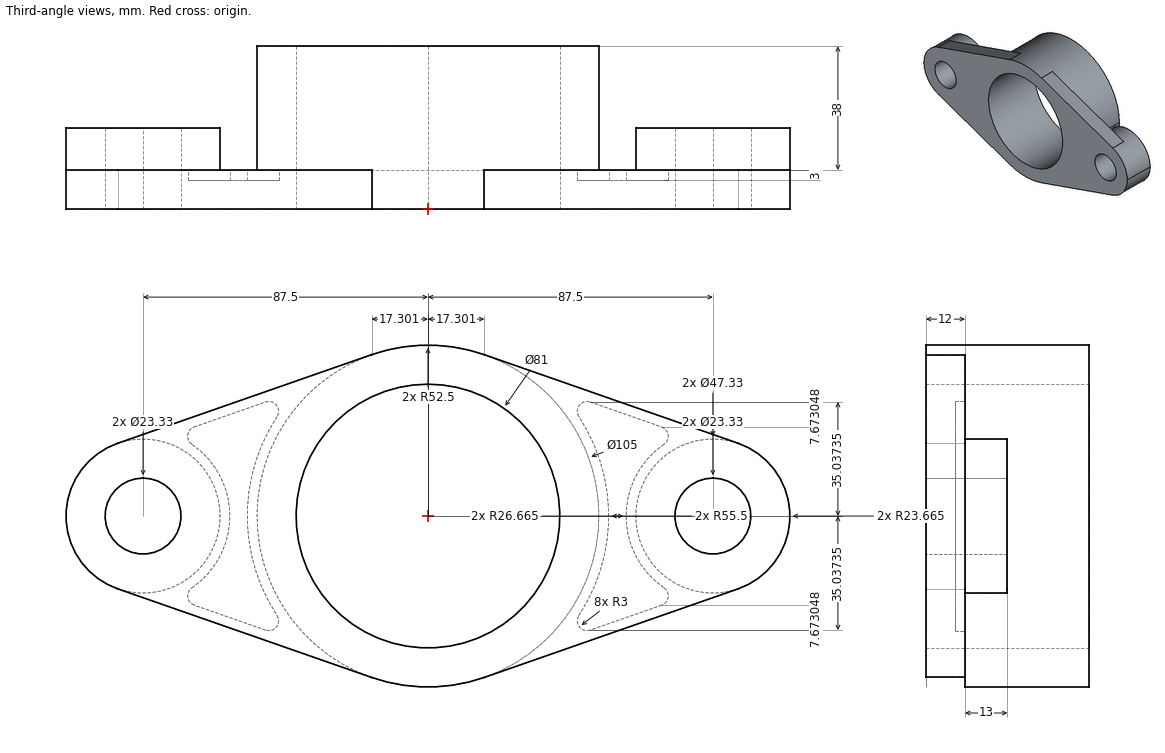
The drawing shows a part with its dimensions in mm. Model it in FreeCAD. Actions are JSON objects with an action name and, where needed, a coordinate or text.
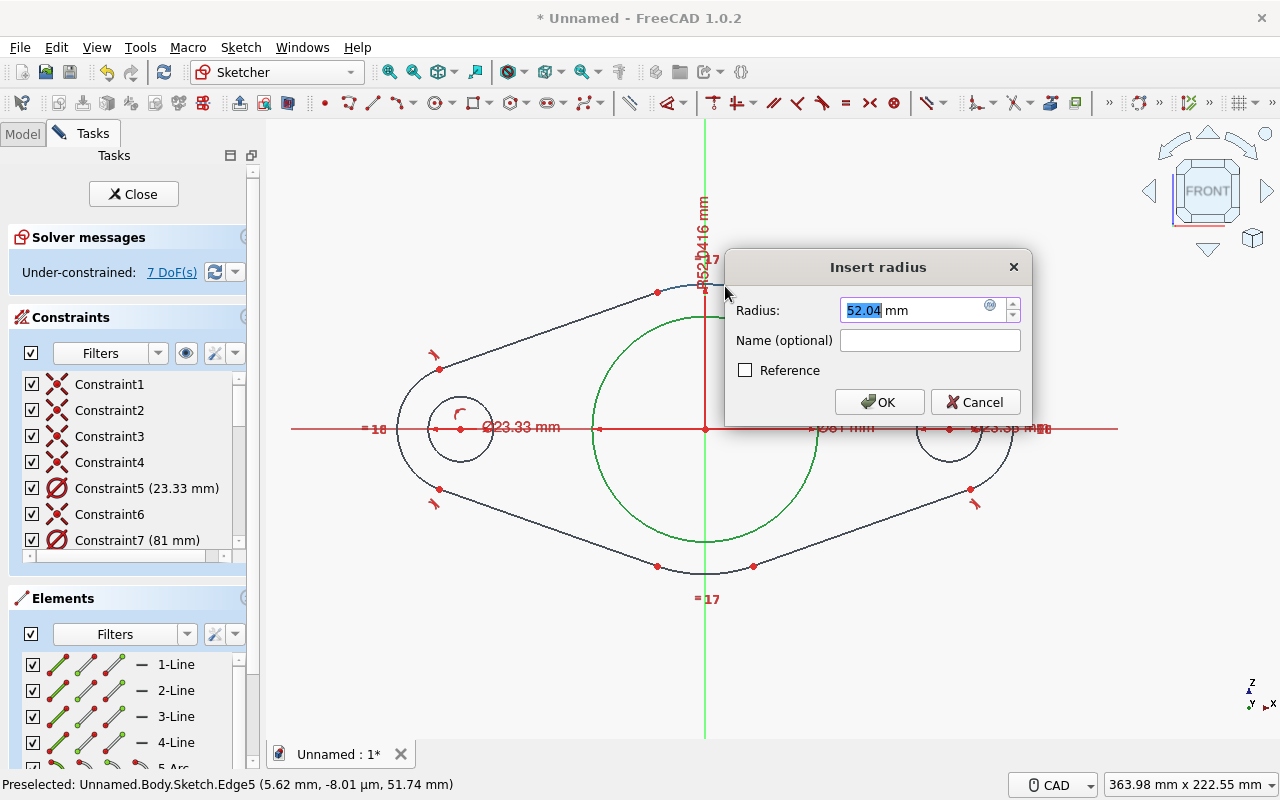
{"action": "type", "text": "52.5"}
{"action": "key", "text": "Return"}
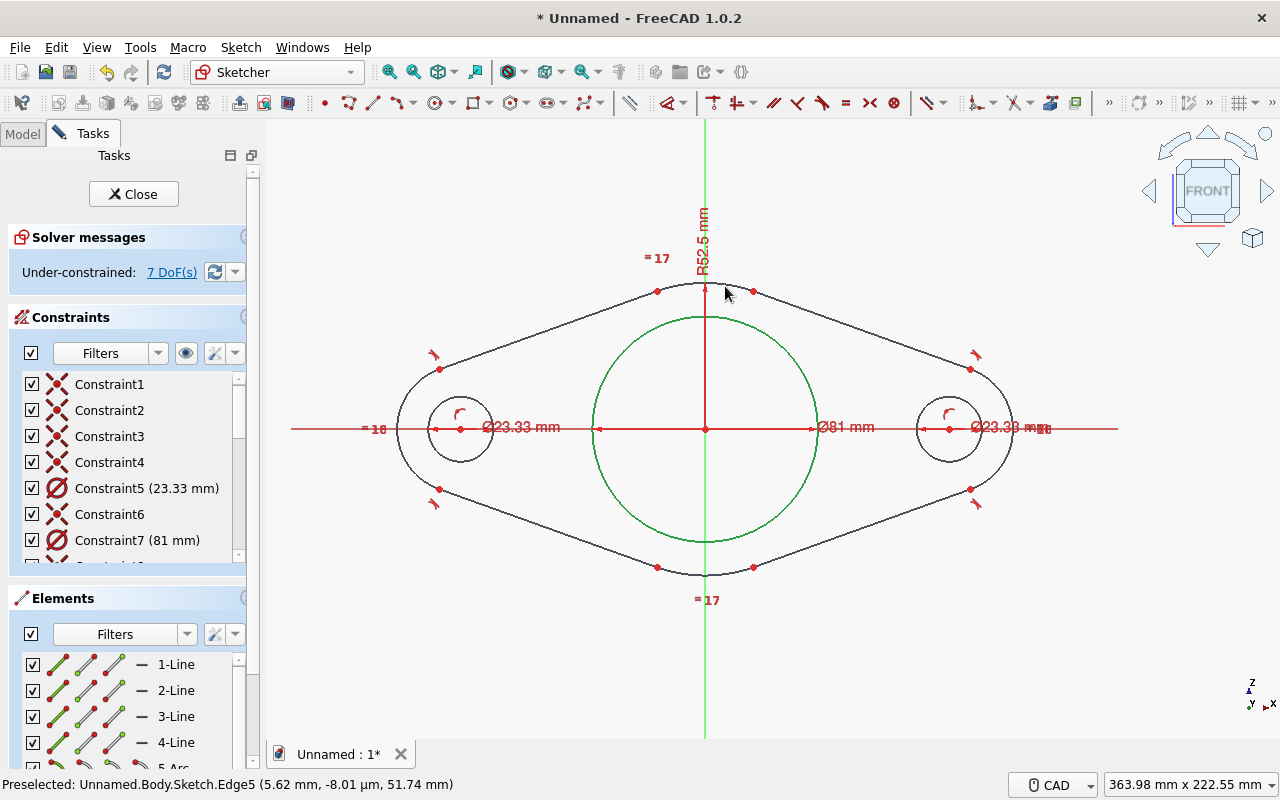
{"action": "left_click", "coordinate": [1005, 459]}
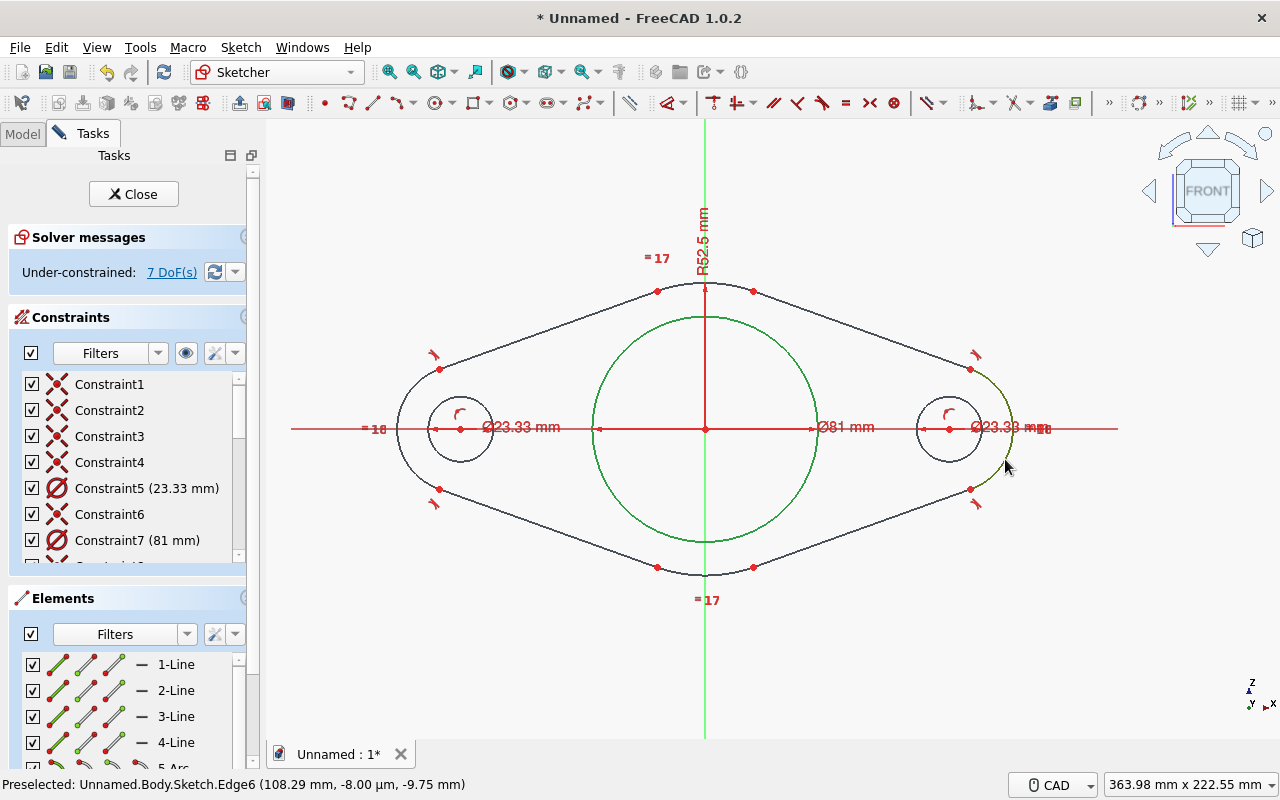
{"action": "left_click", "coordinate": [686, 104]}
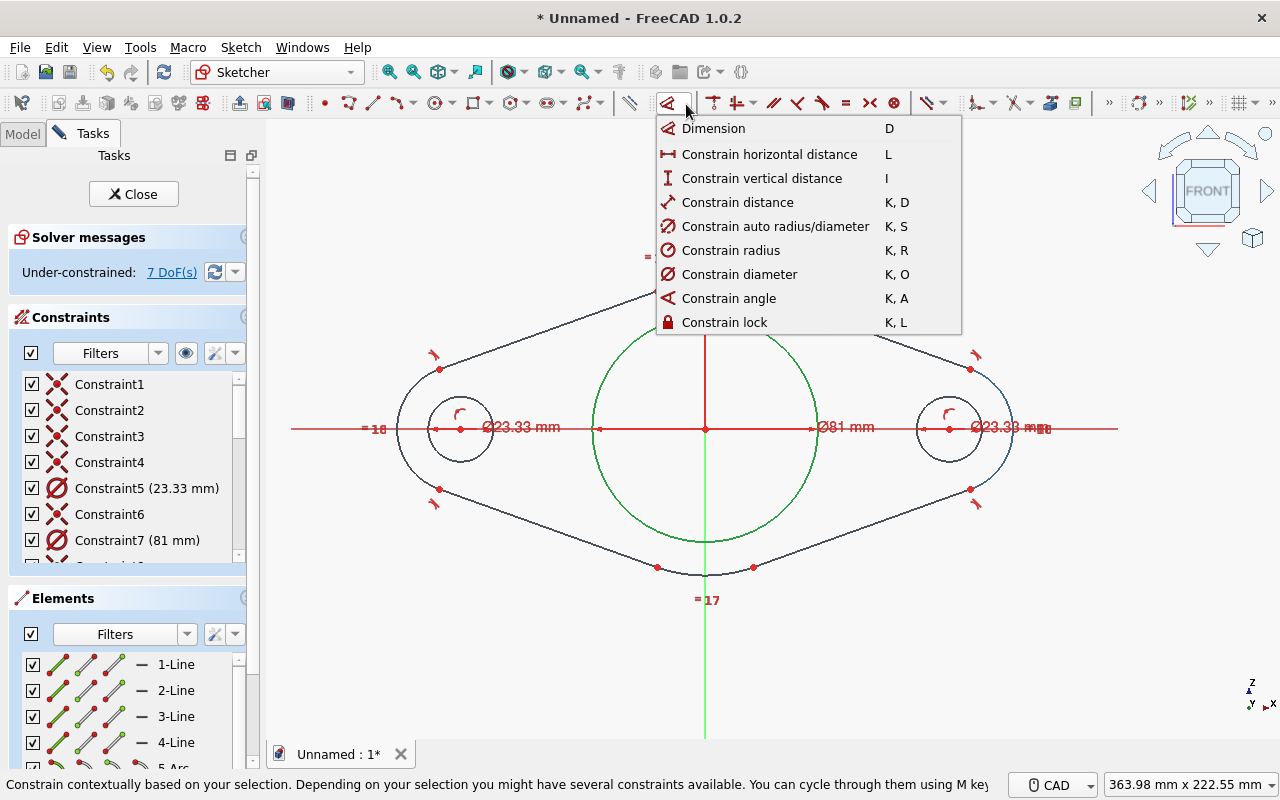
{"action": "left_click", "coordinate": [809, 250]}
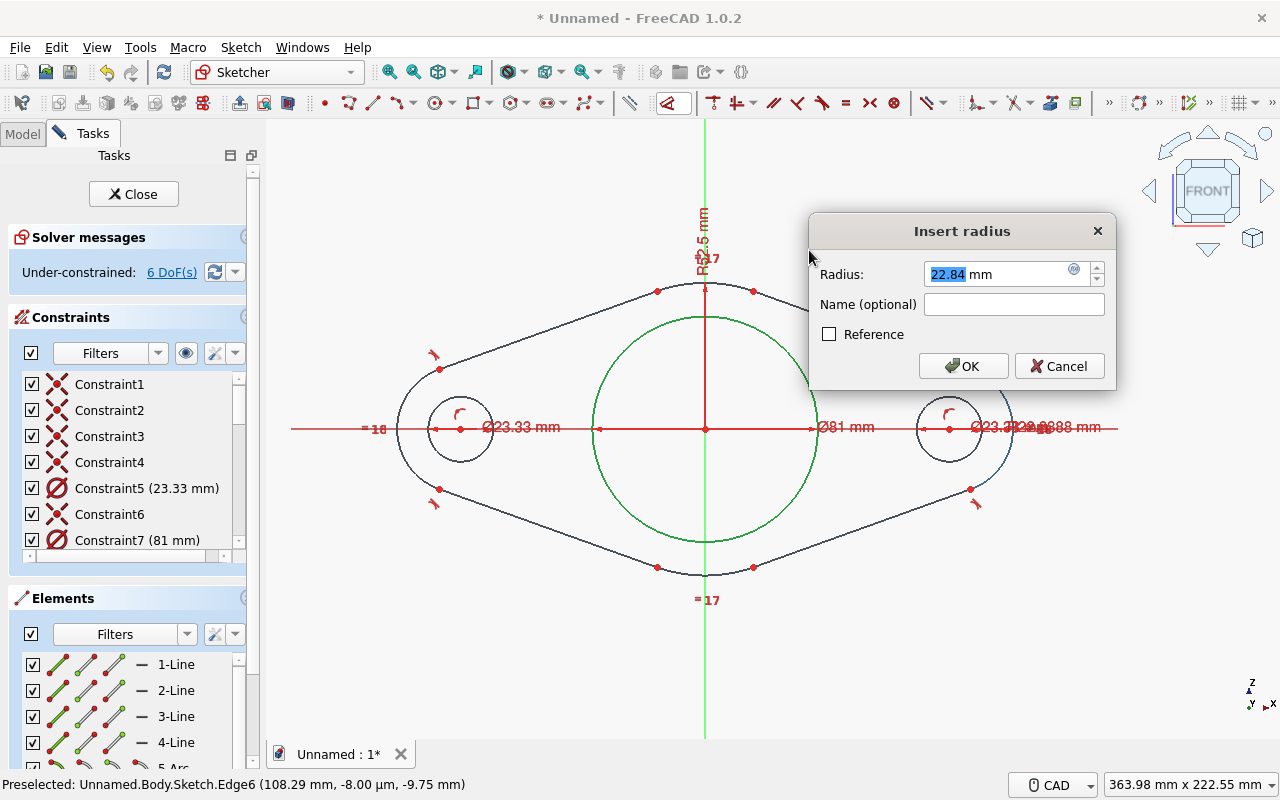
{"action": "type", "text": "23.665"}
{"action": "key", "text": "Return"}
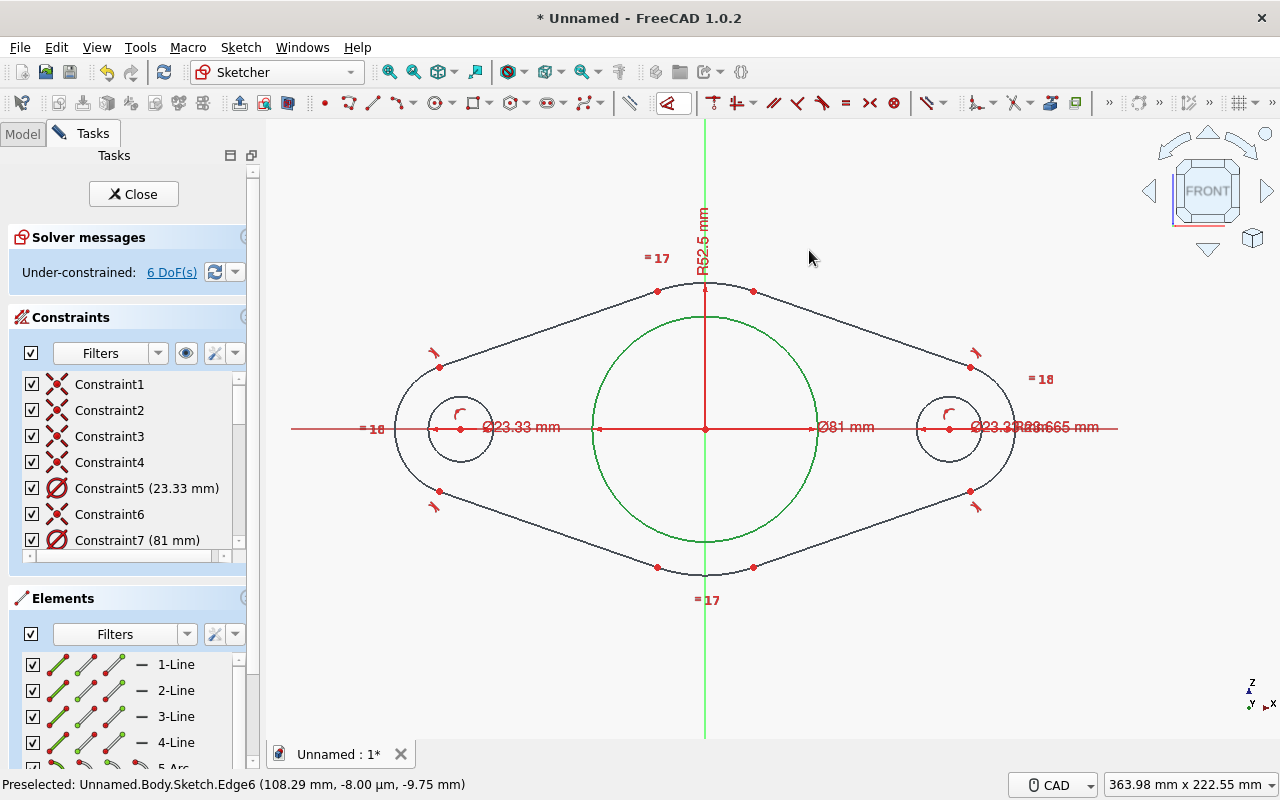
{"action": "left_click", "coordinate": [461, 429]}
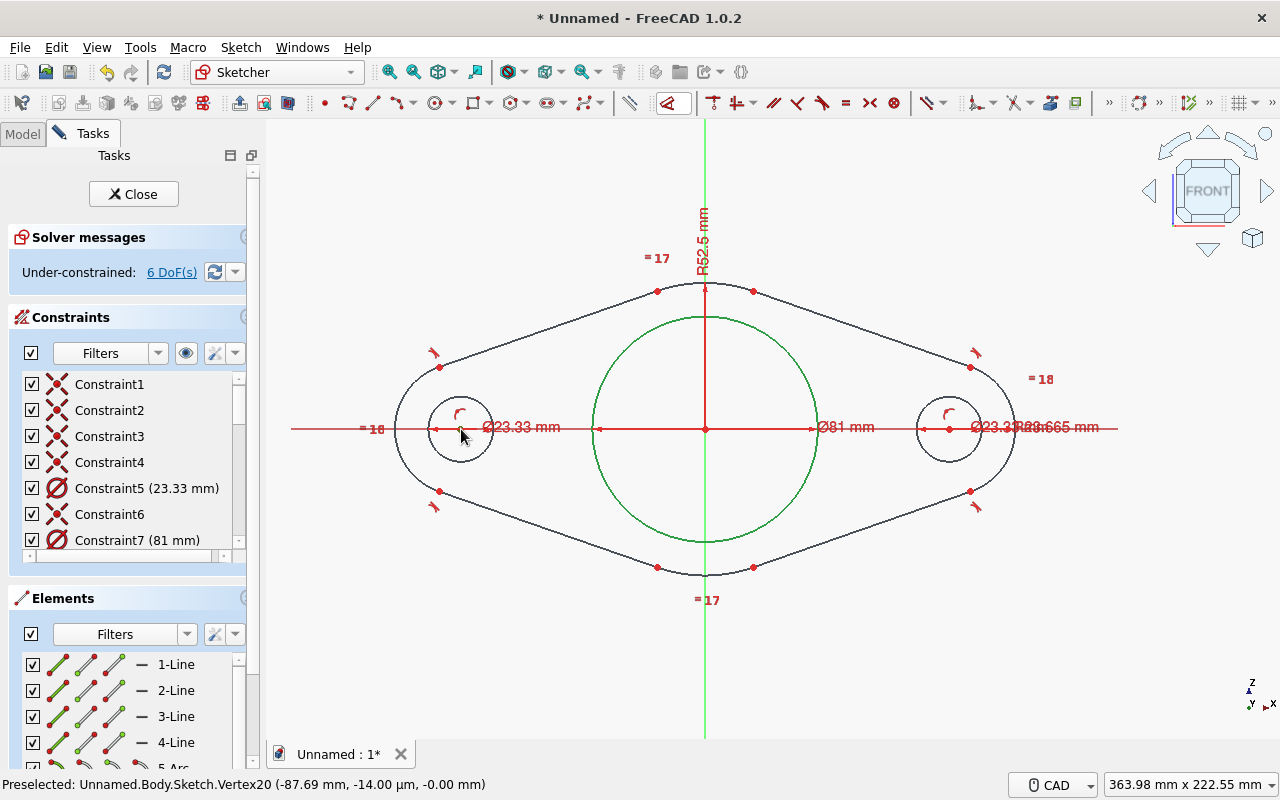
{"action": "key", "text": "l"}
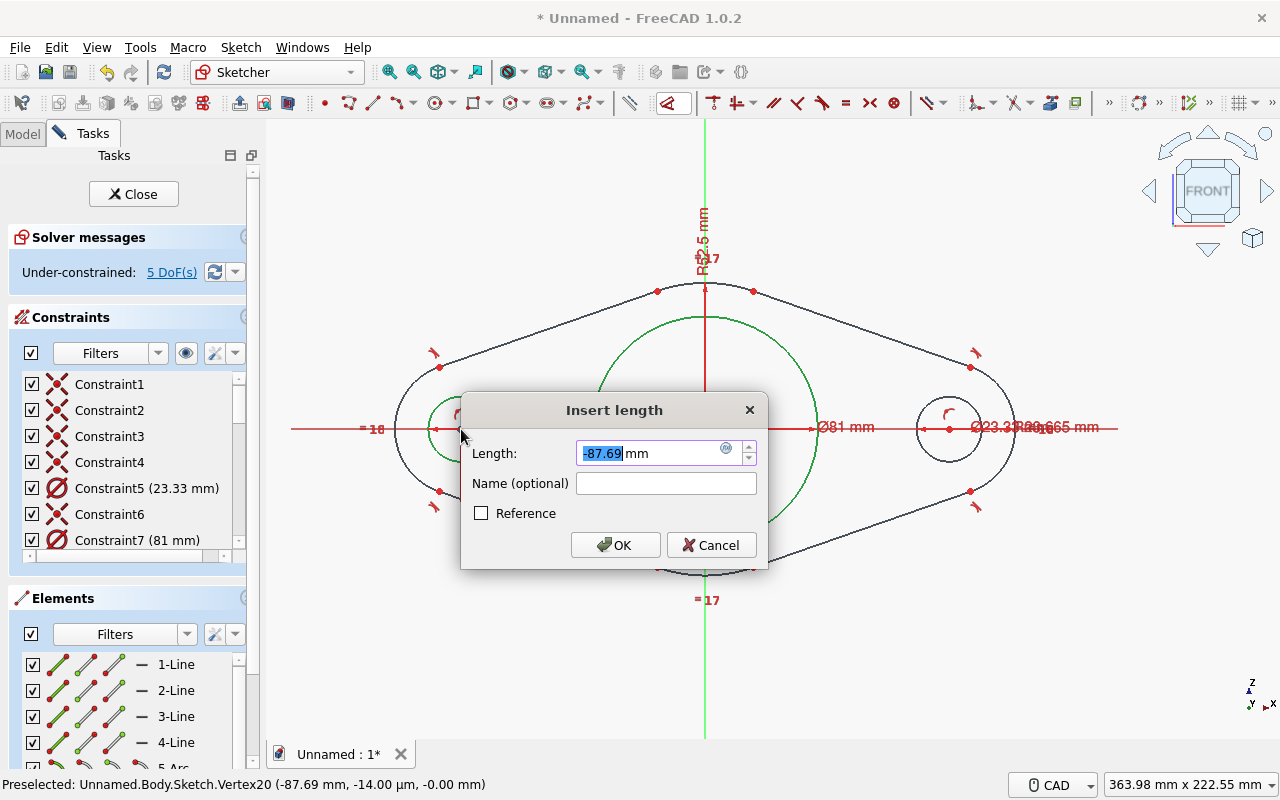
{"action": "type", "text": "-87.5"}
{"action": "key", "text": "Return"}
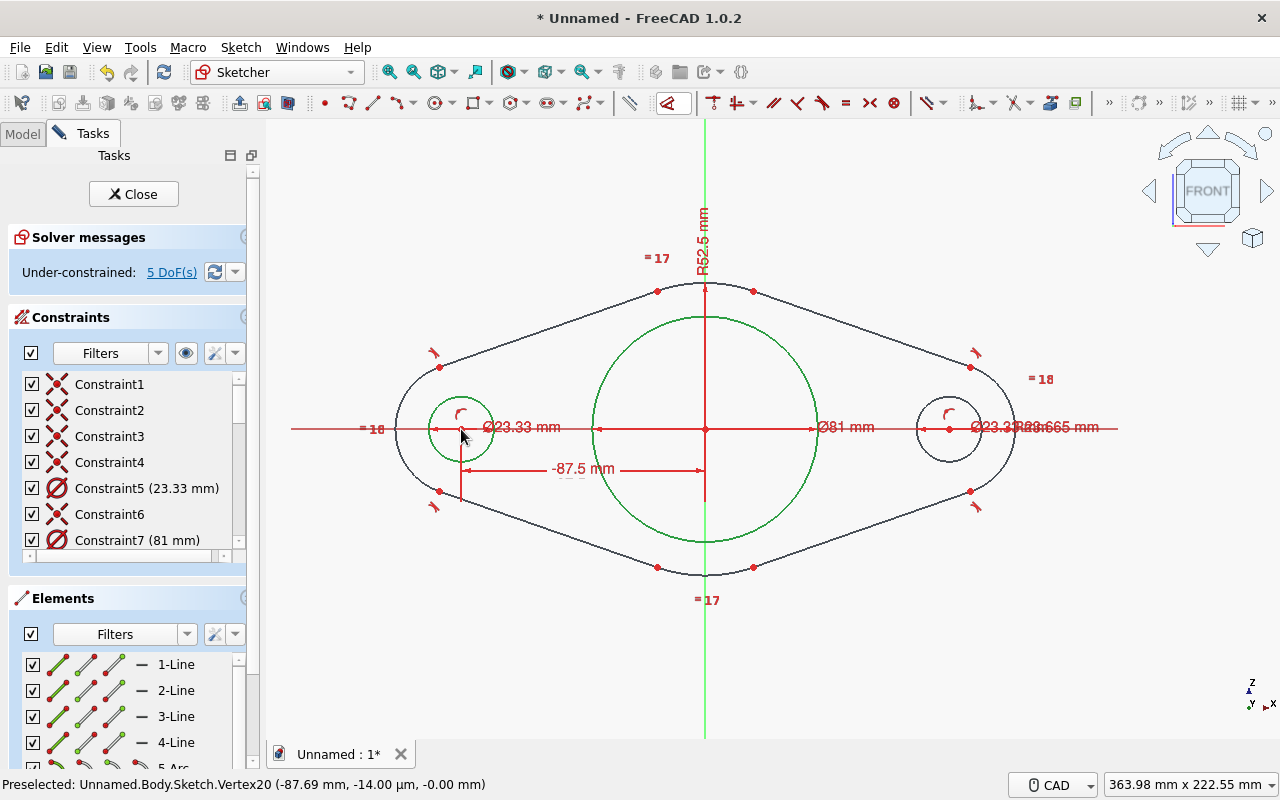
{"action": "left_click", "coordinate": [949, 429]}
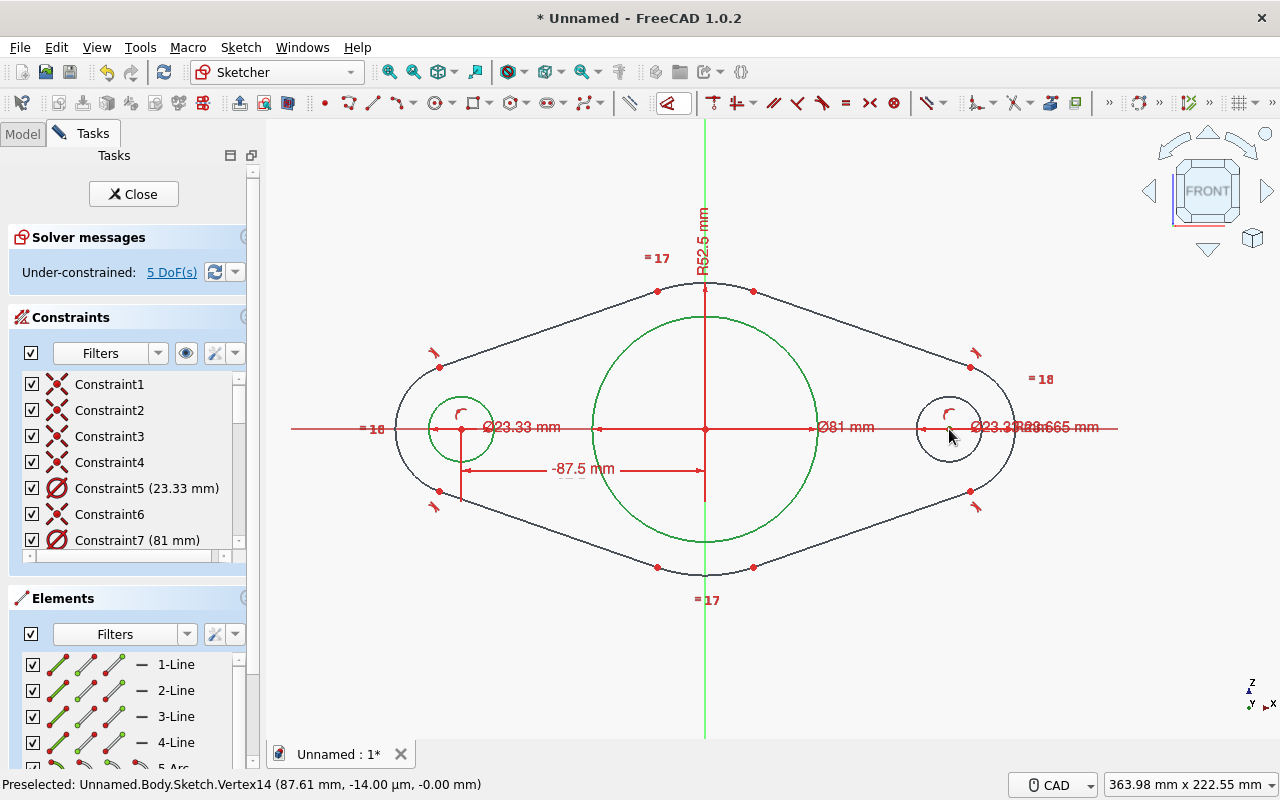
{"action": "left_click", "coordinate": [686, 104]}